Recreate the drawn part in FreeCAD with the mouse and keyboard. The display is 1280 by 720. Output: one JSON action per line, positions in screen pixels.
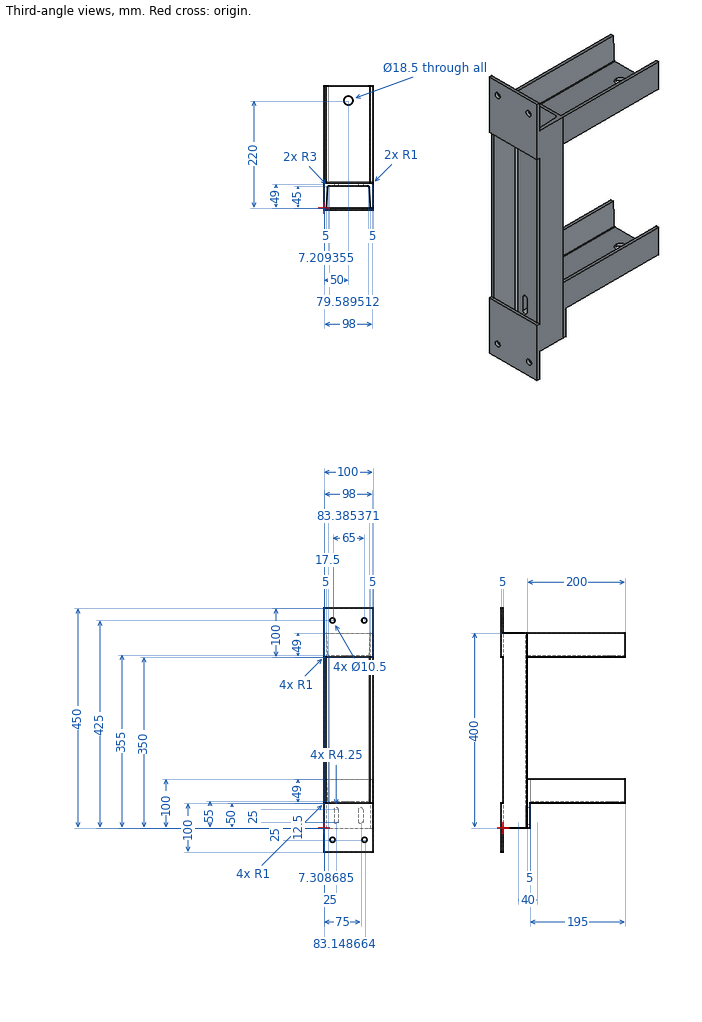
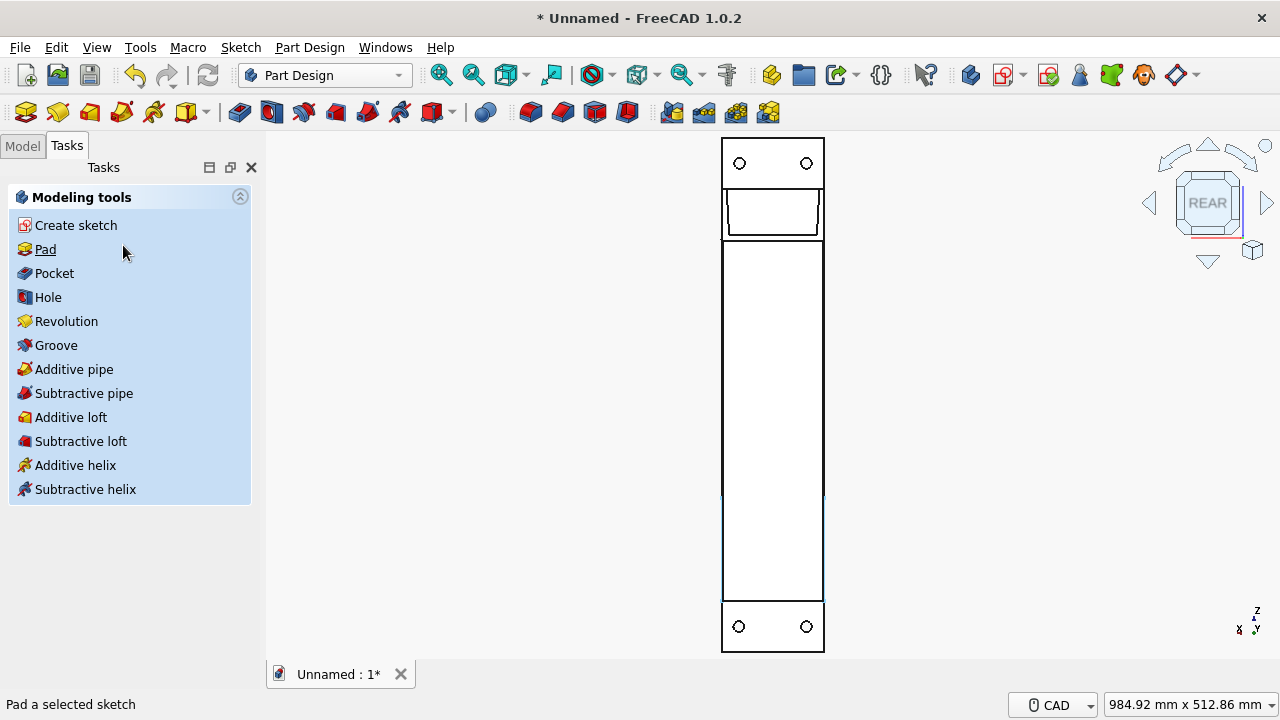
{"action": "left_click", "coordinate": [26, 112]}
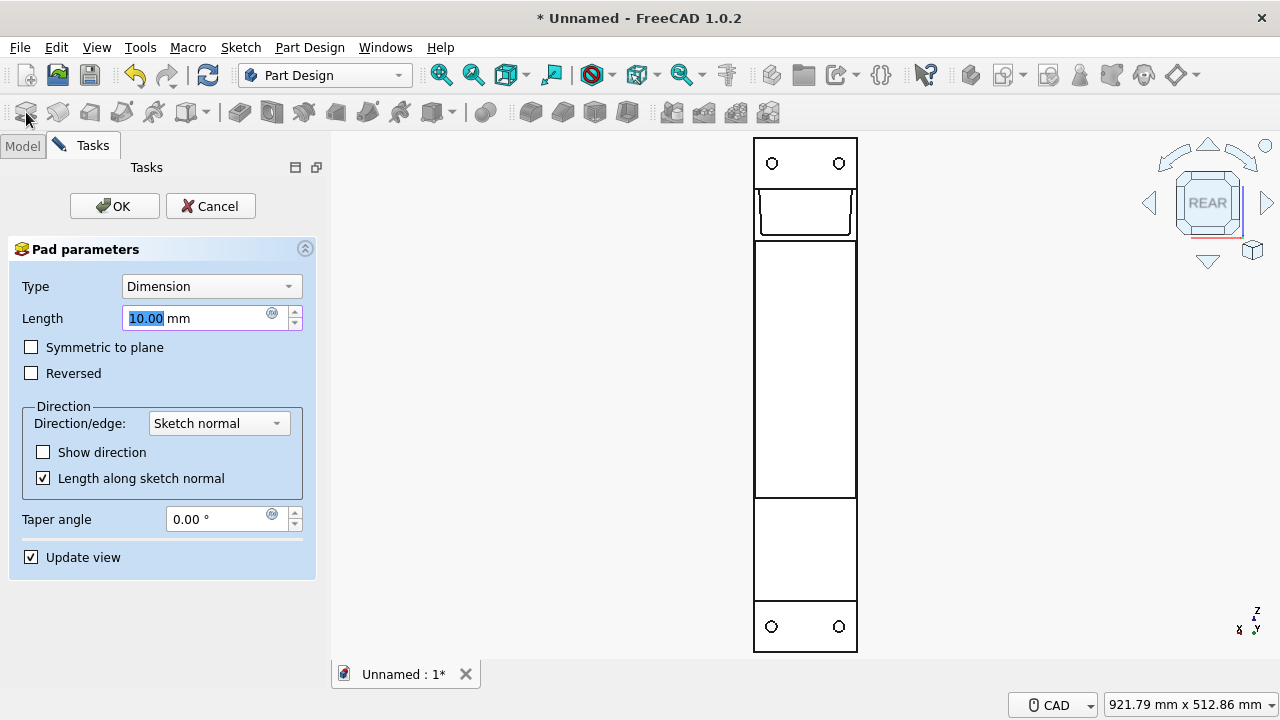
{"action": "type", "text": "5"}
{"action": "key", "text": "Tab"}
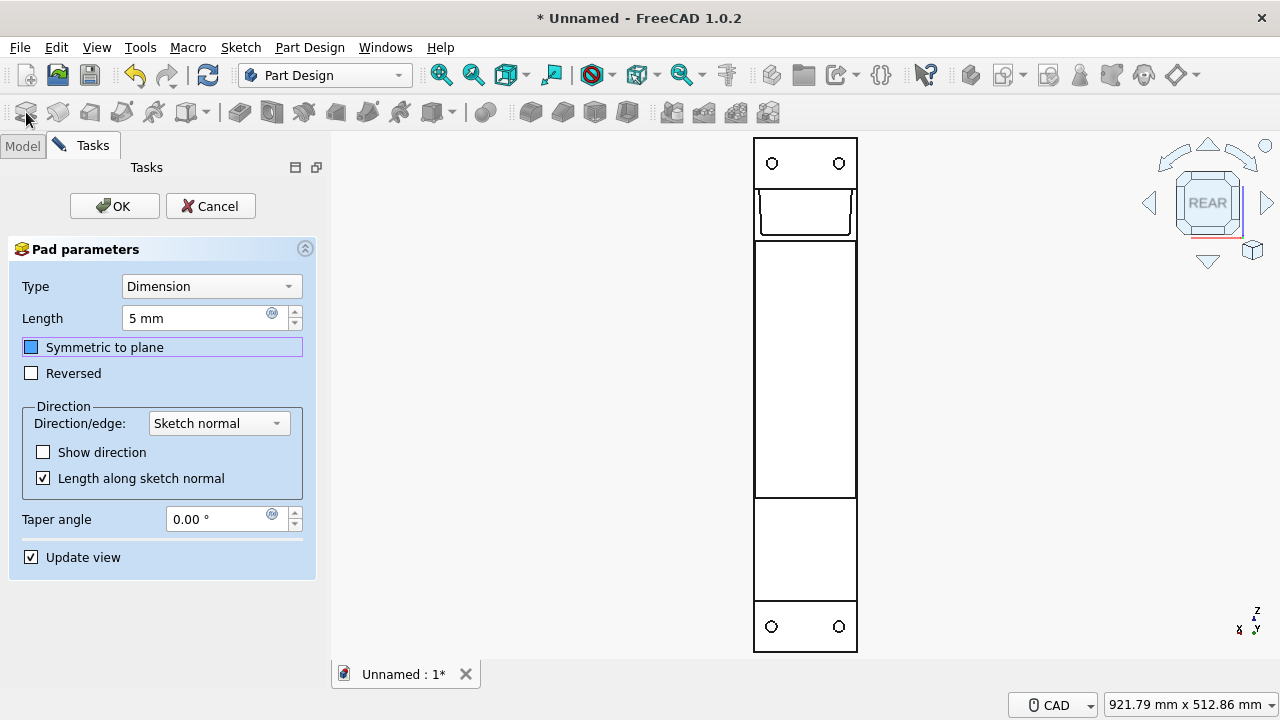
{"action": "left_click", "coordinate": [115, 206]}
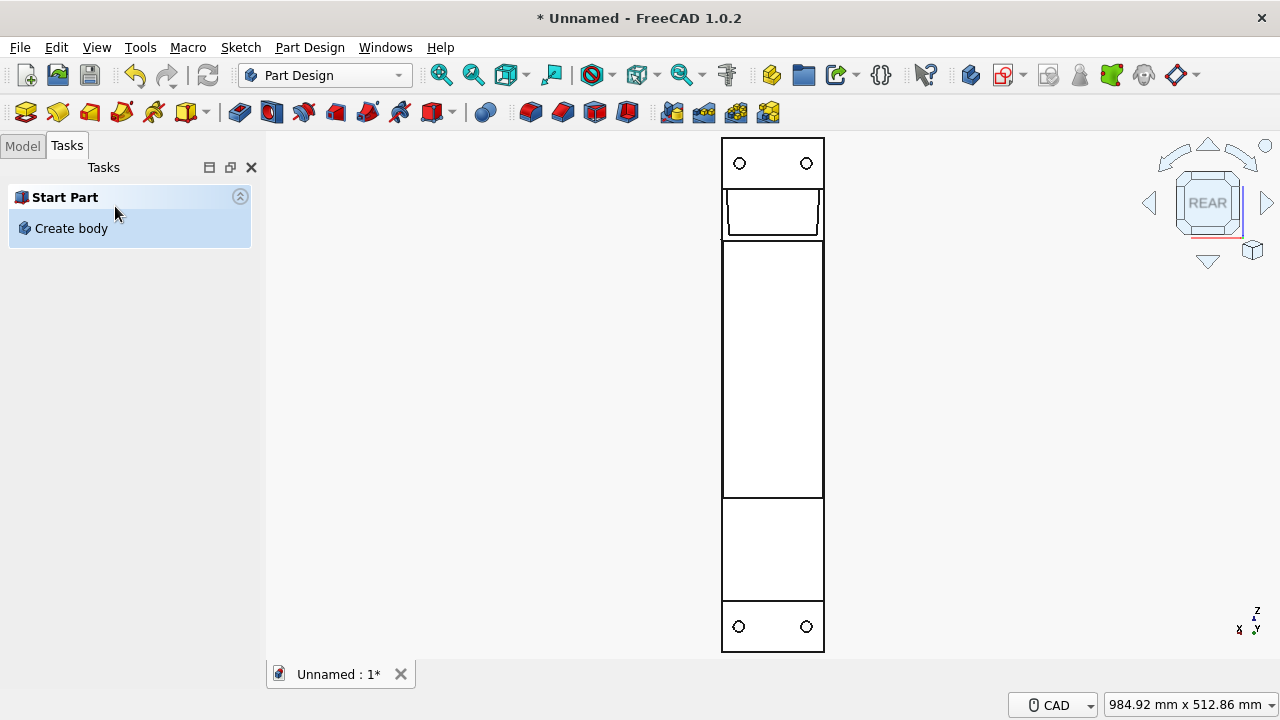
{"action": "left_click", "coordinate": [773, 548]}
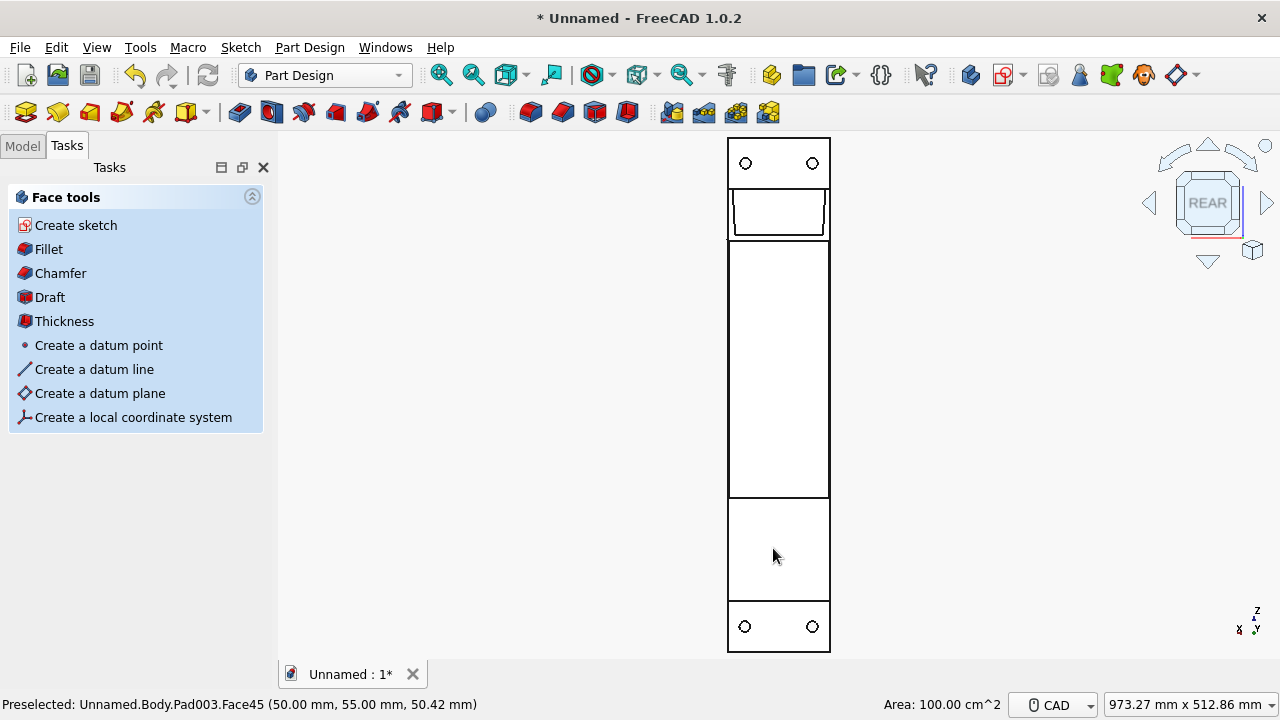
{"action": "left_click", "coordinate": [1004, 76]}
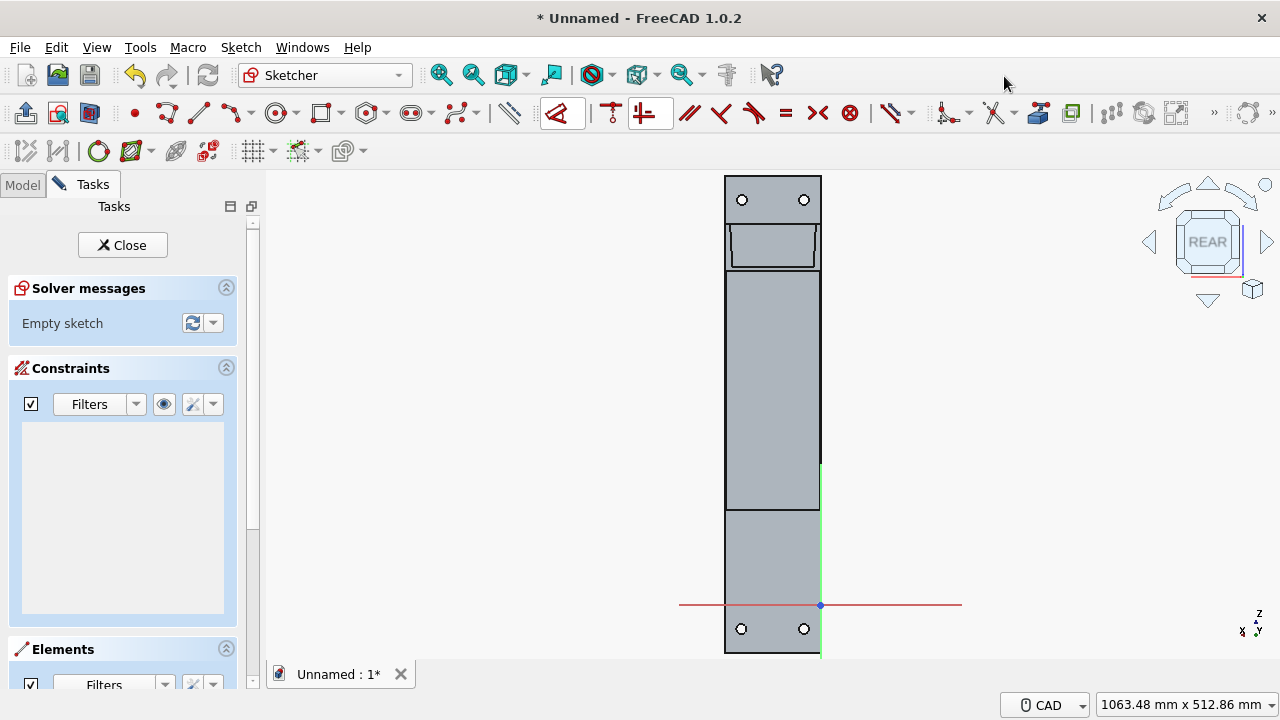
{"action": "scroll", "coordinate": [803, 619], "scroll_direction": "up", "scroll_amount": 6}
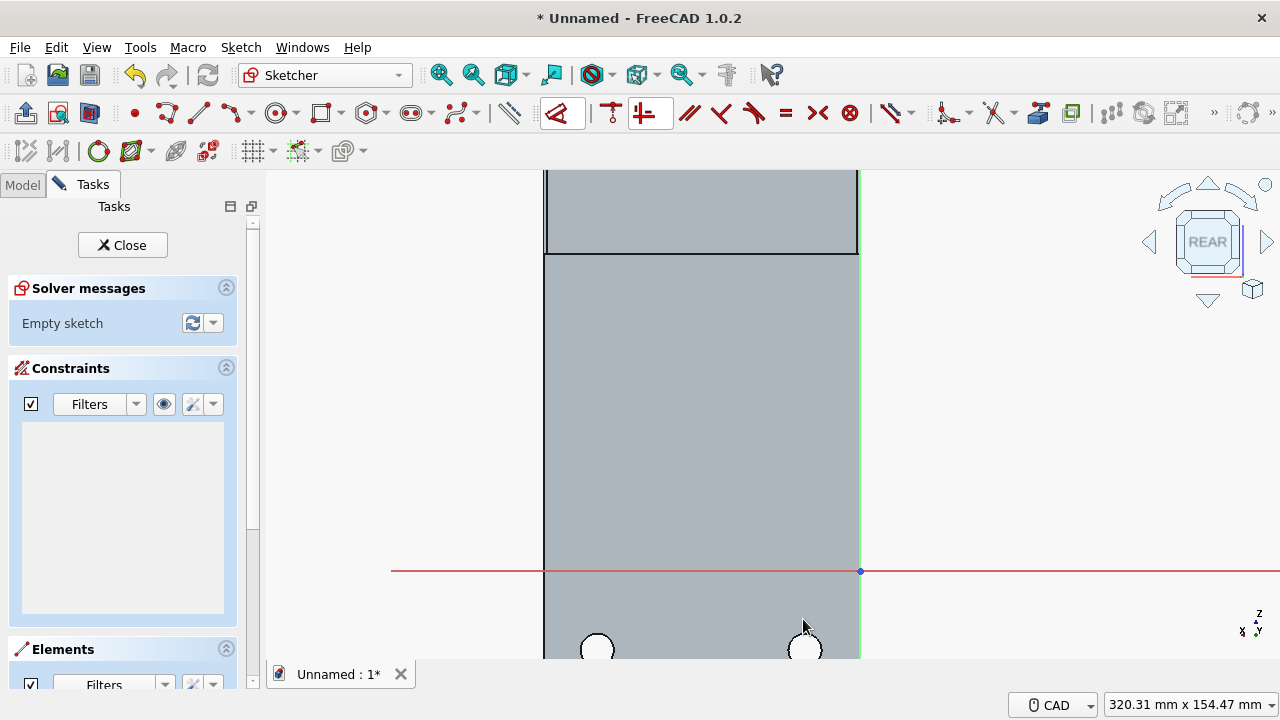
{"action": "left_click", "coordinate": [200, 114]}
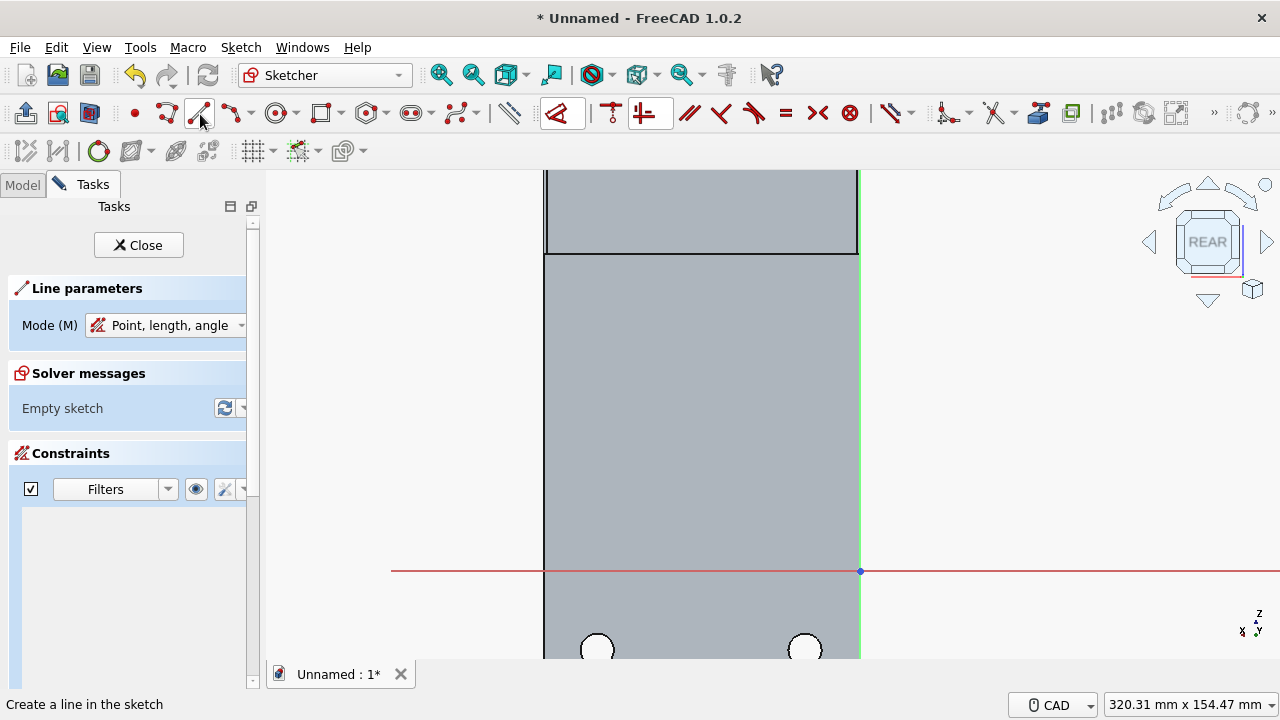
{"action": "left_click", "coordinate": [547, 413]}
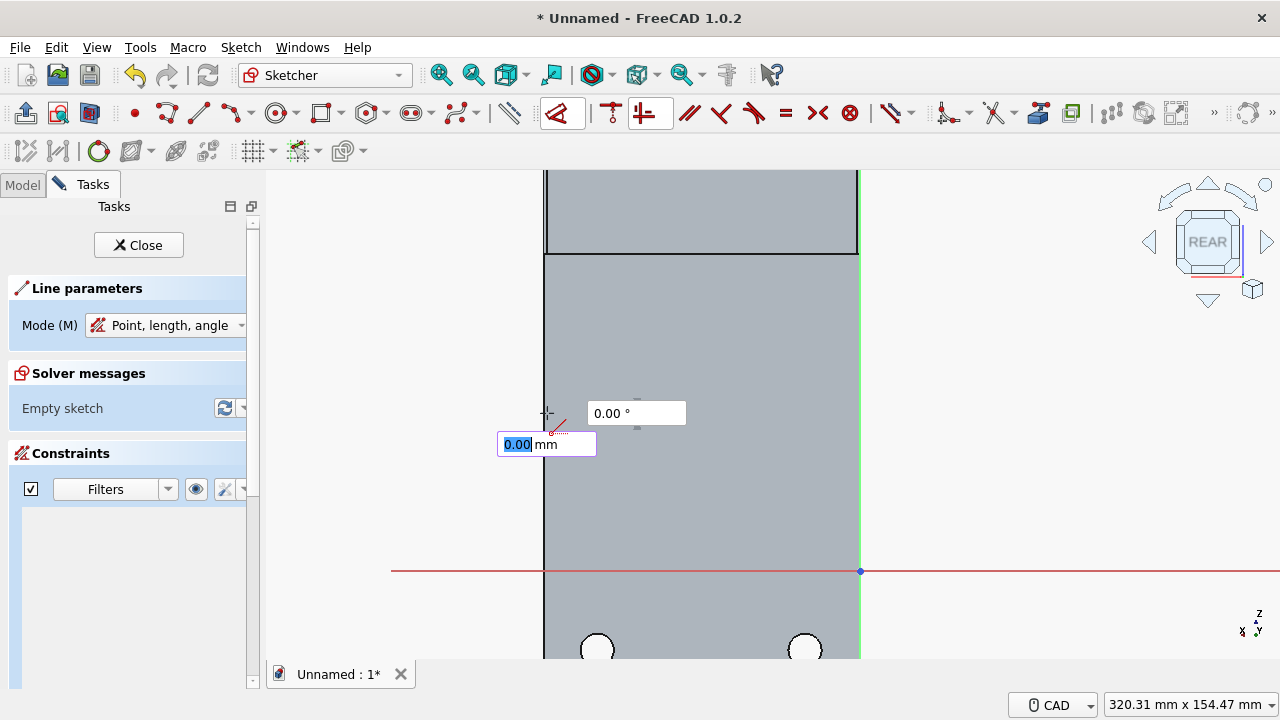
{"action": "scroll", "coordinate": [857, 413], "scroll_direction": "up", "scroll_amount": 9}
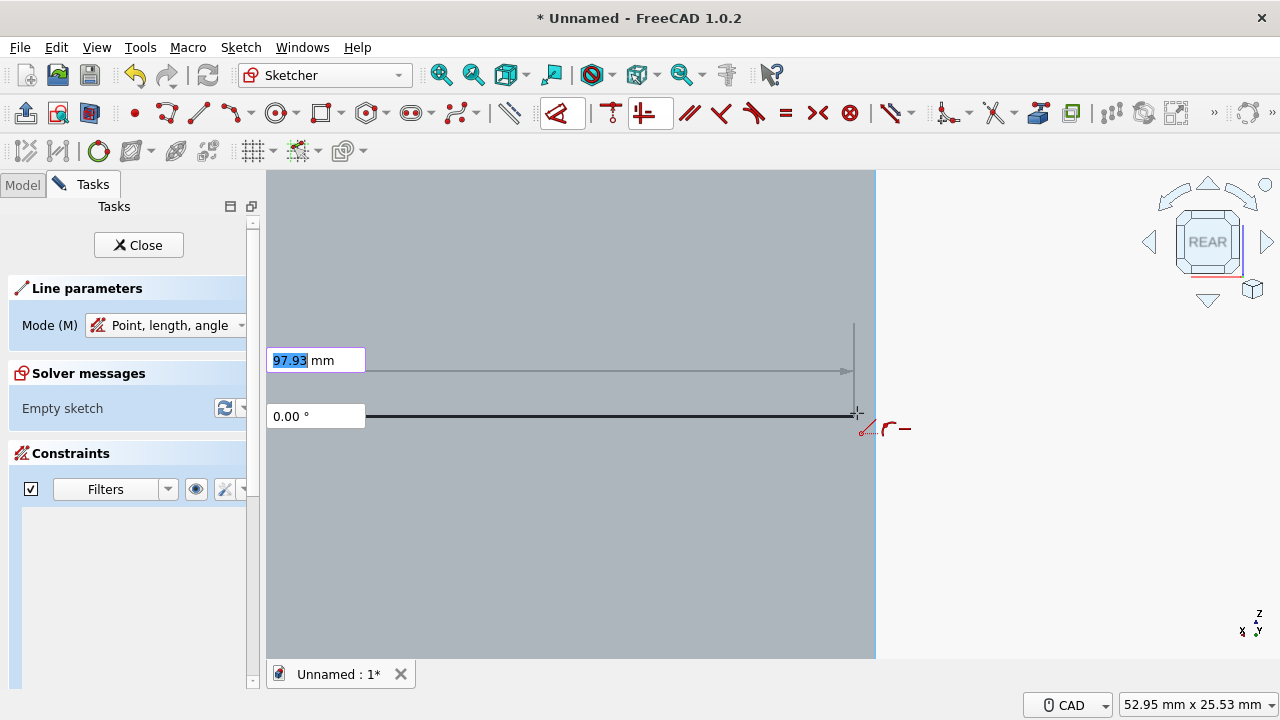
{"action": "left_click", "coordinate": [856, 410]}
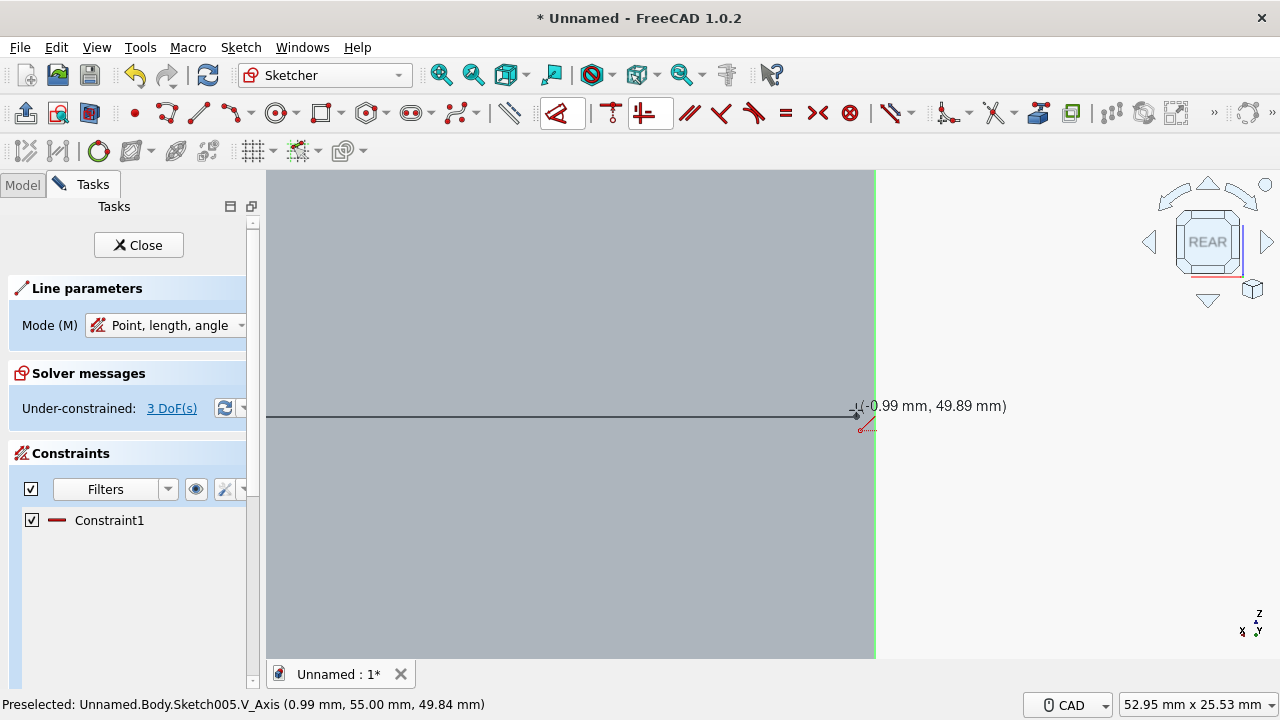
{"action": "left_click", "coordinate": [168, 114]}